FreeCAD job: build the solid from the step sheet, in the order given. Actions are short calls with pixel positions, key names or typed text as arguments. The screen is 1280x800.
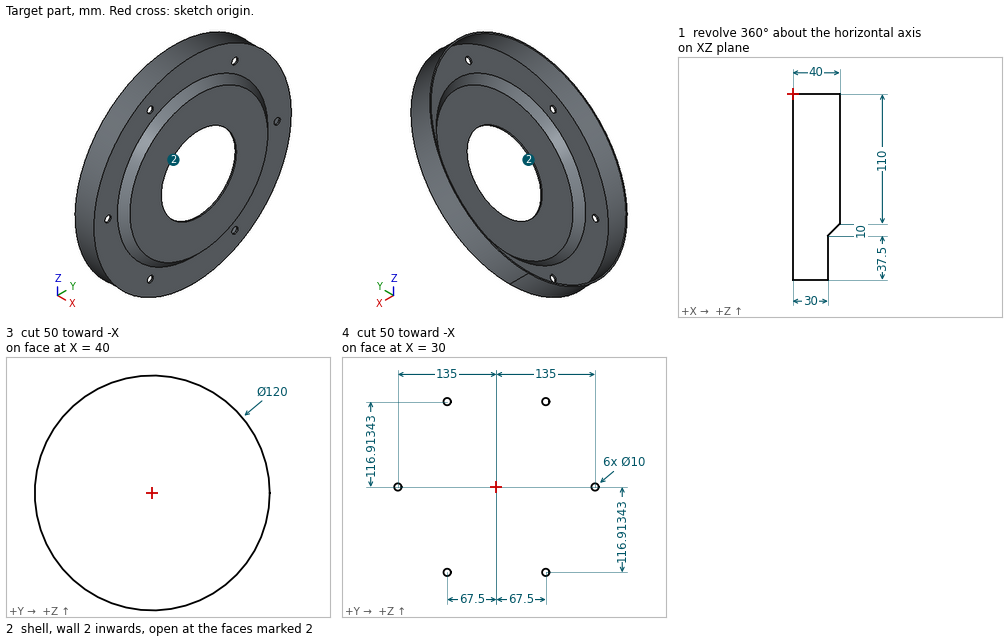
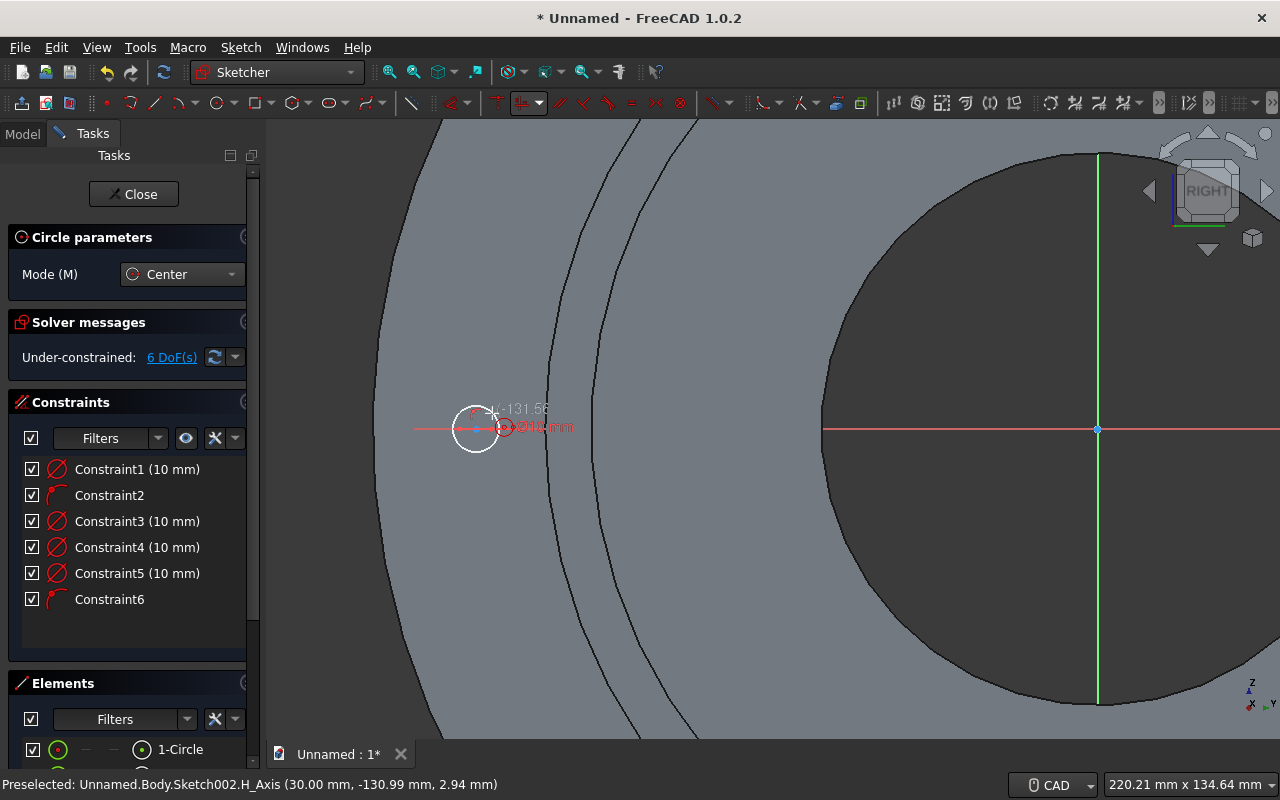
scroll(476, 429, down, 5)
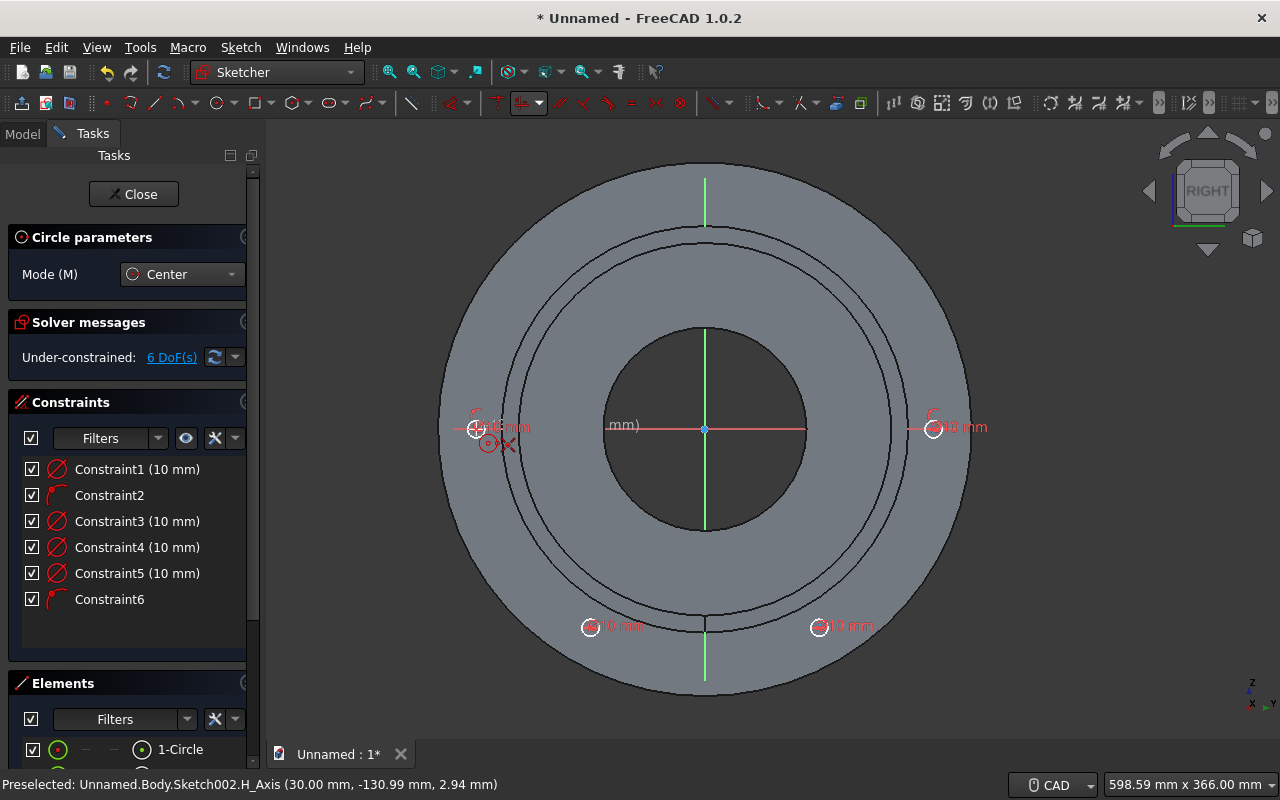
scroll(591, 231, up, 5)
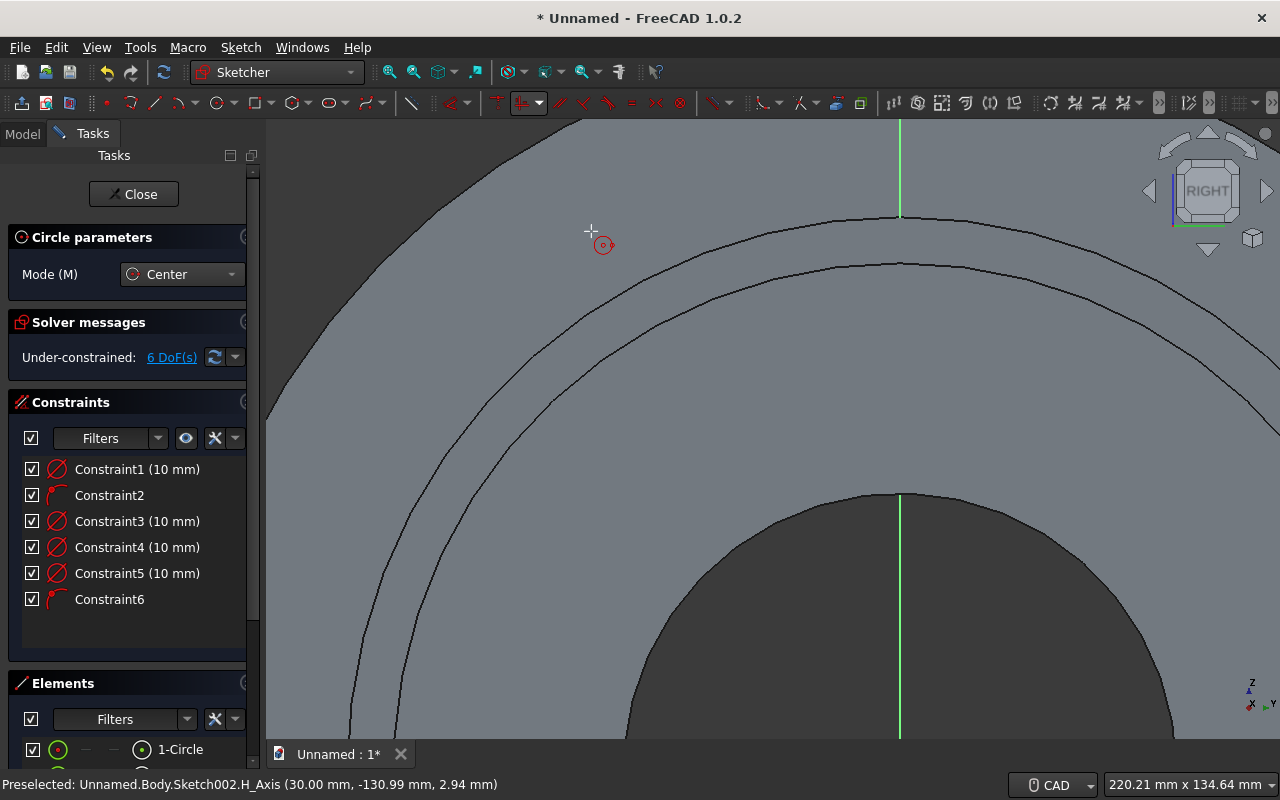
click(589, 231)
move(605, 215)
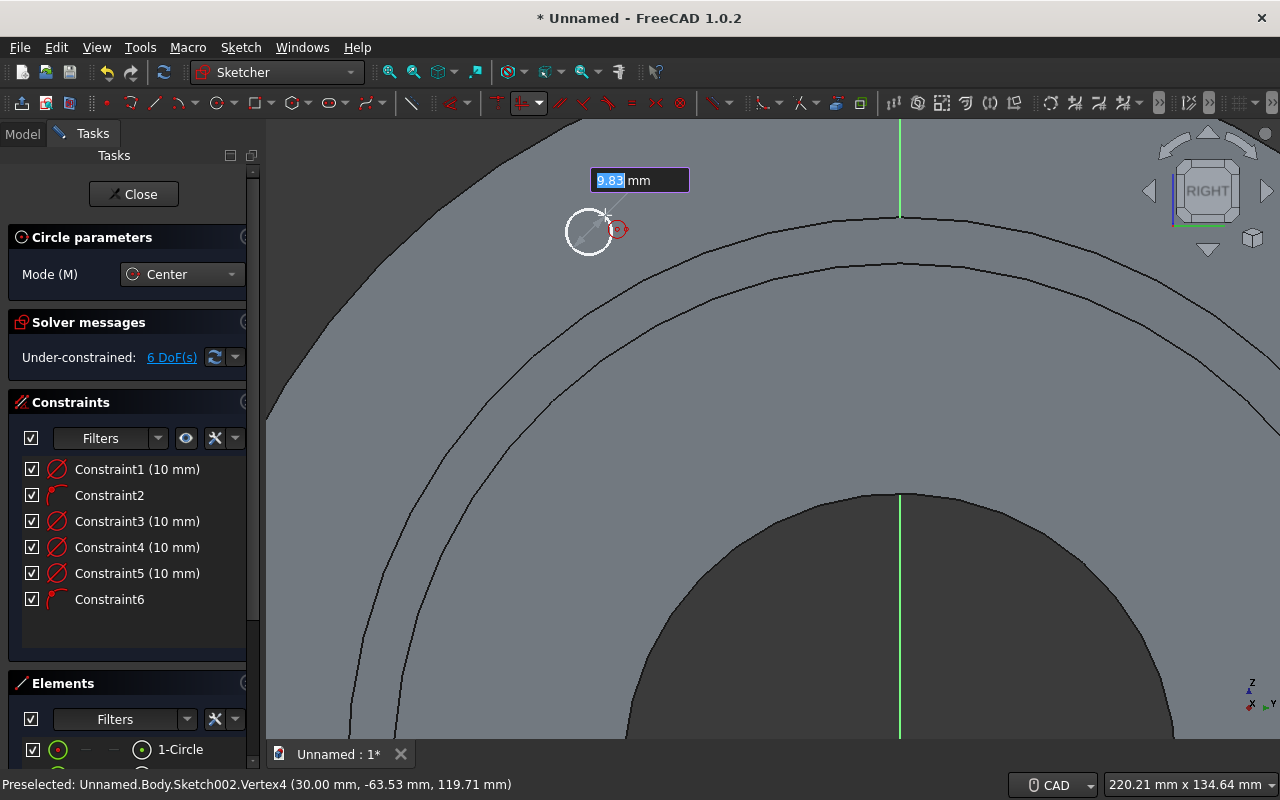
text(10)
key(Return)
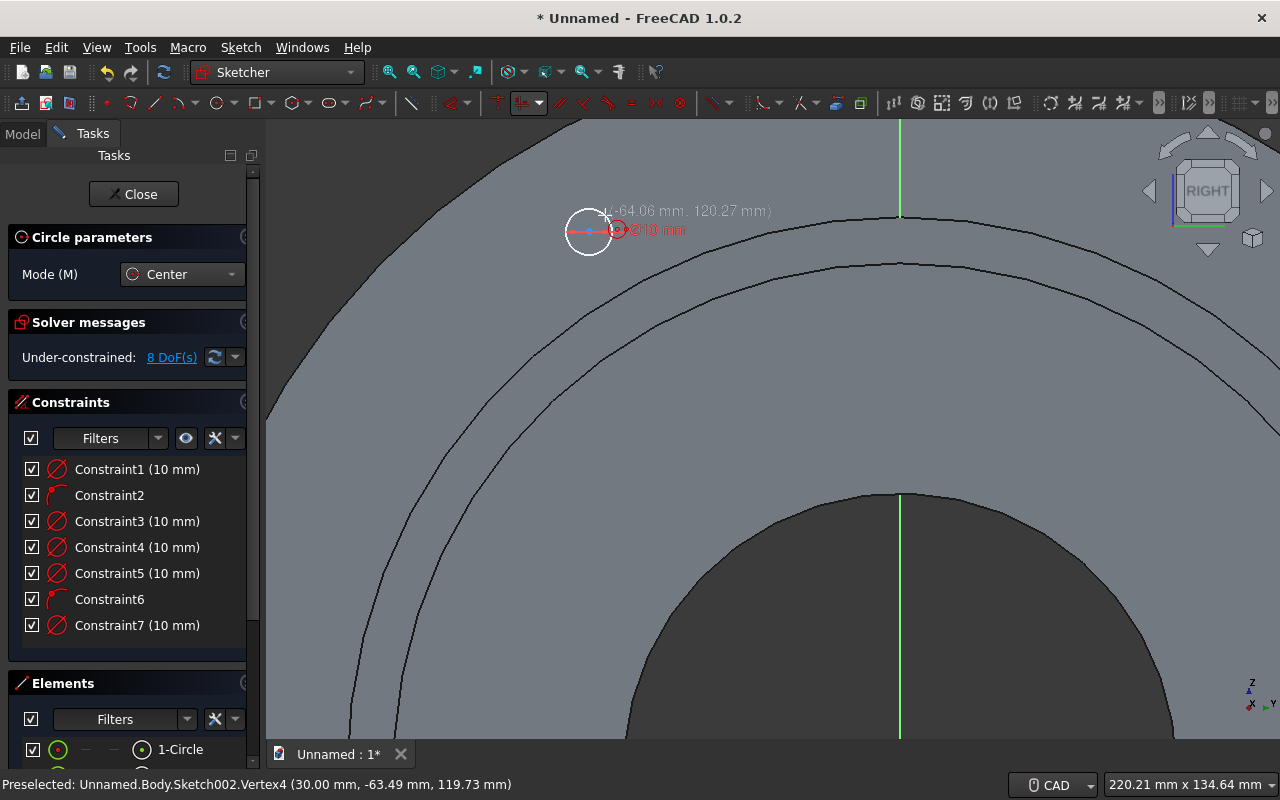
scroll(591, 231, down, 5)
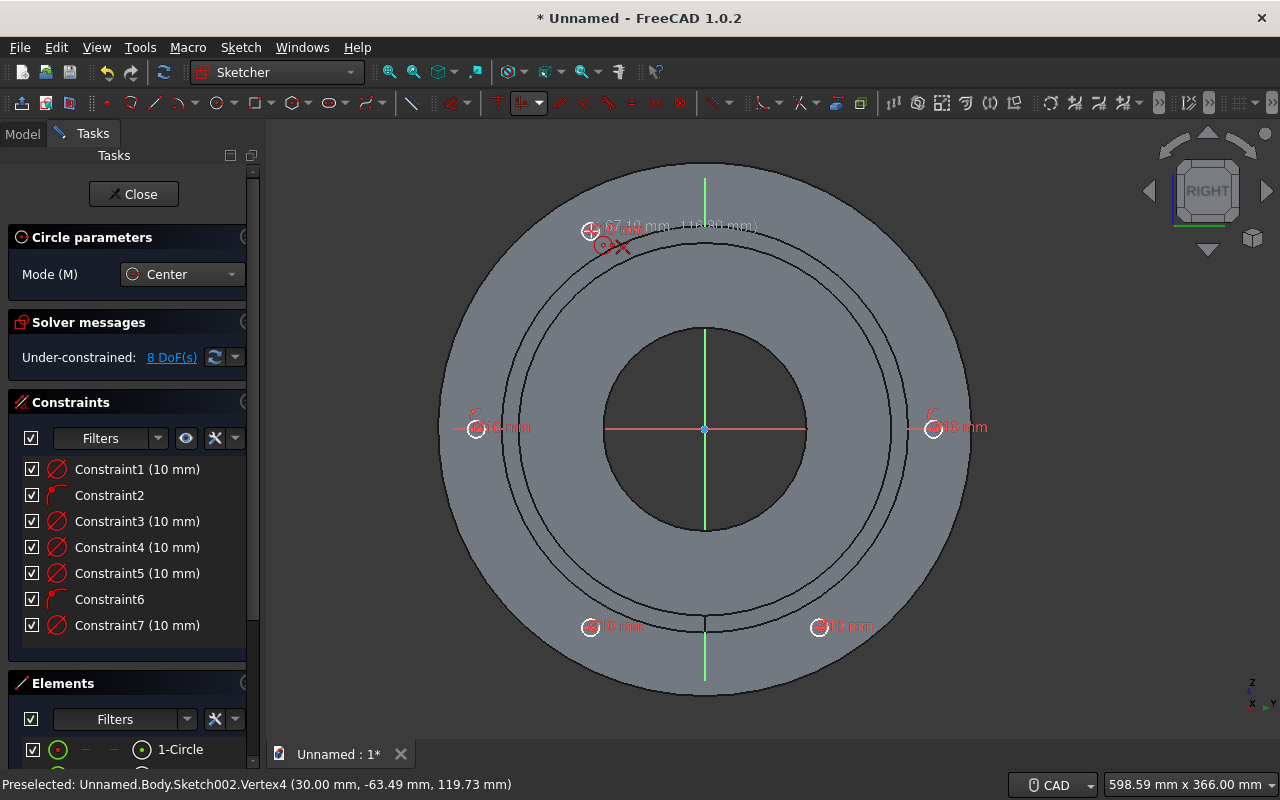
scroll(819, 231, up, 5)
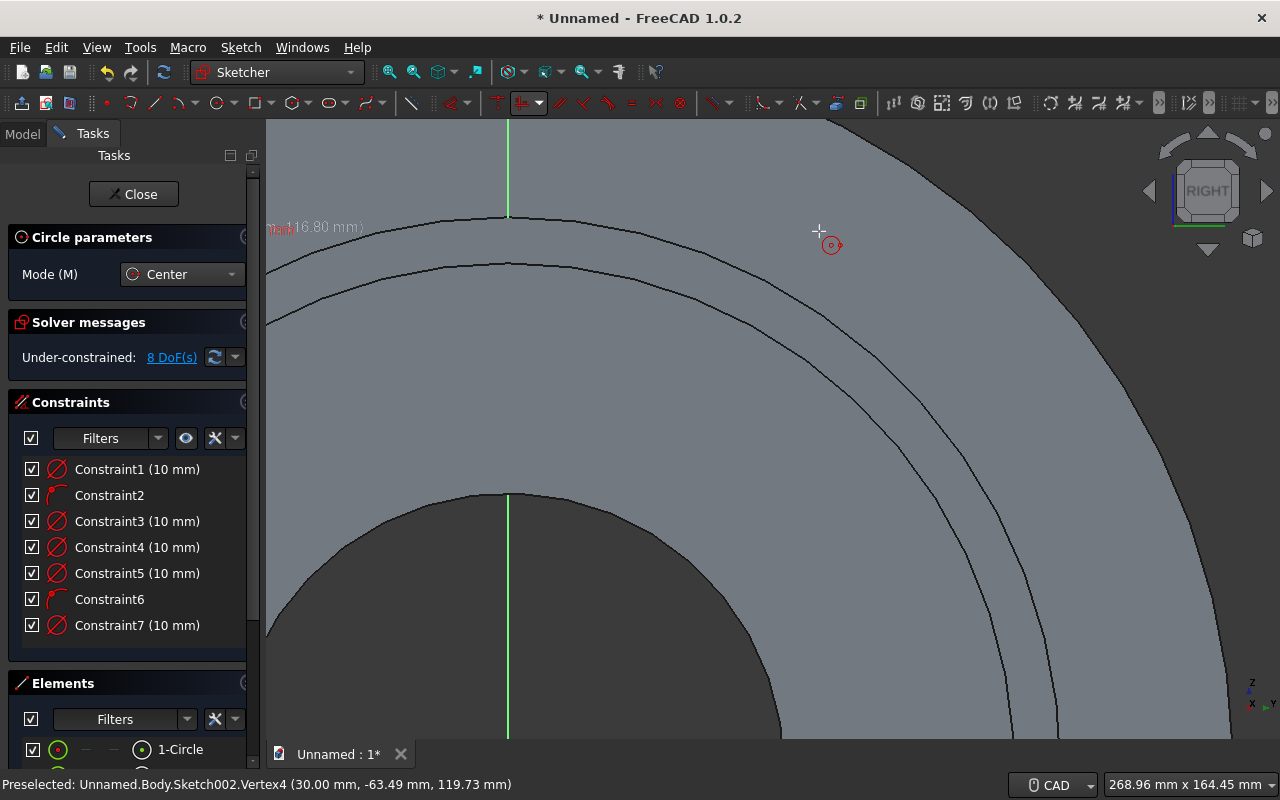
click(819, 231)
move(835, 215)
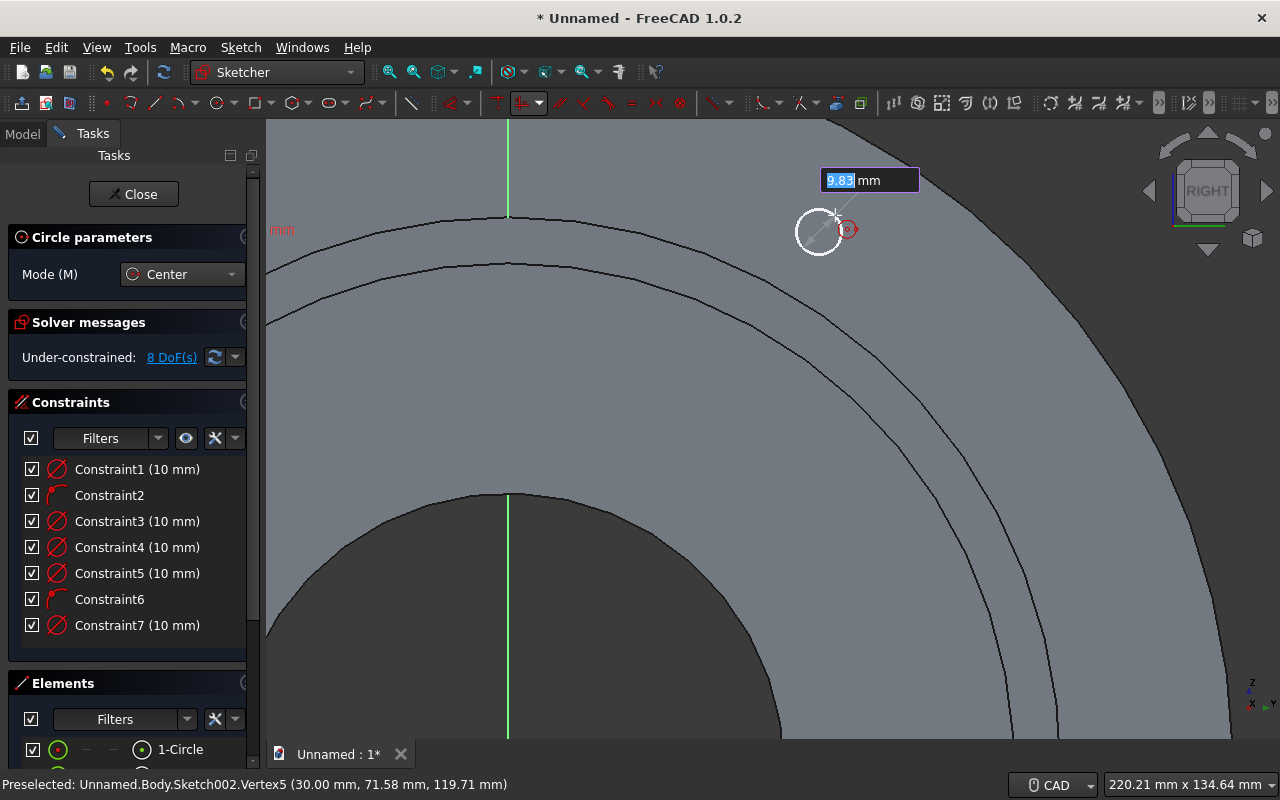
text(10)
key(Return)
key(Escape)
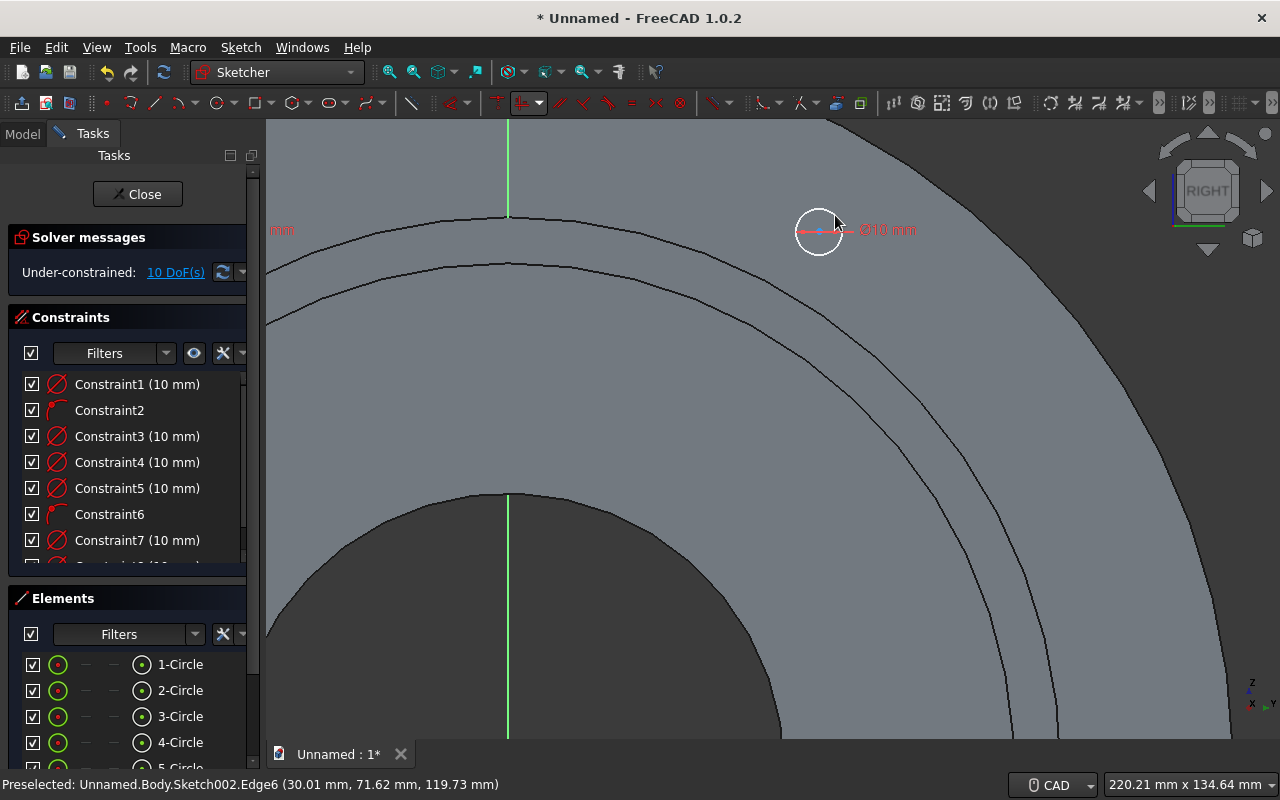
scroll(819, 231, down, 5)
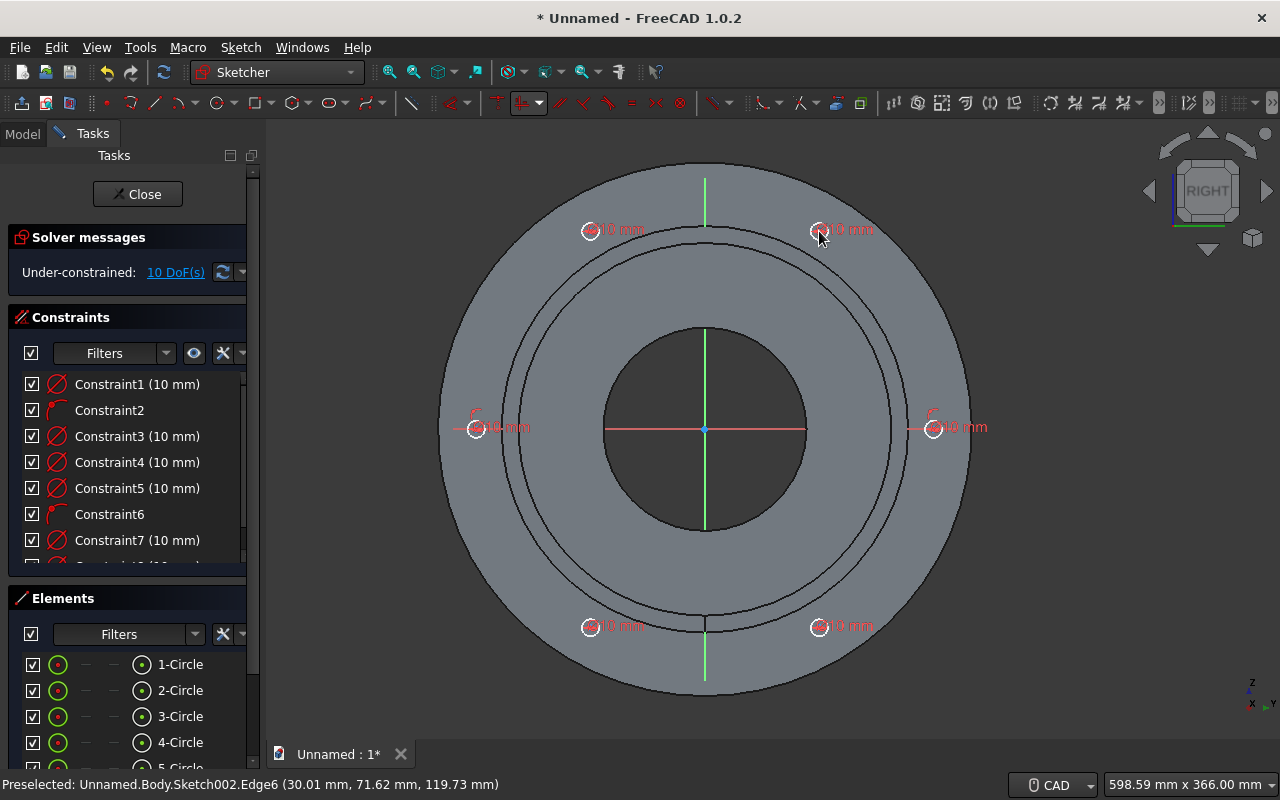
click(819, 628)